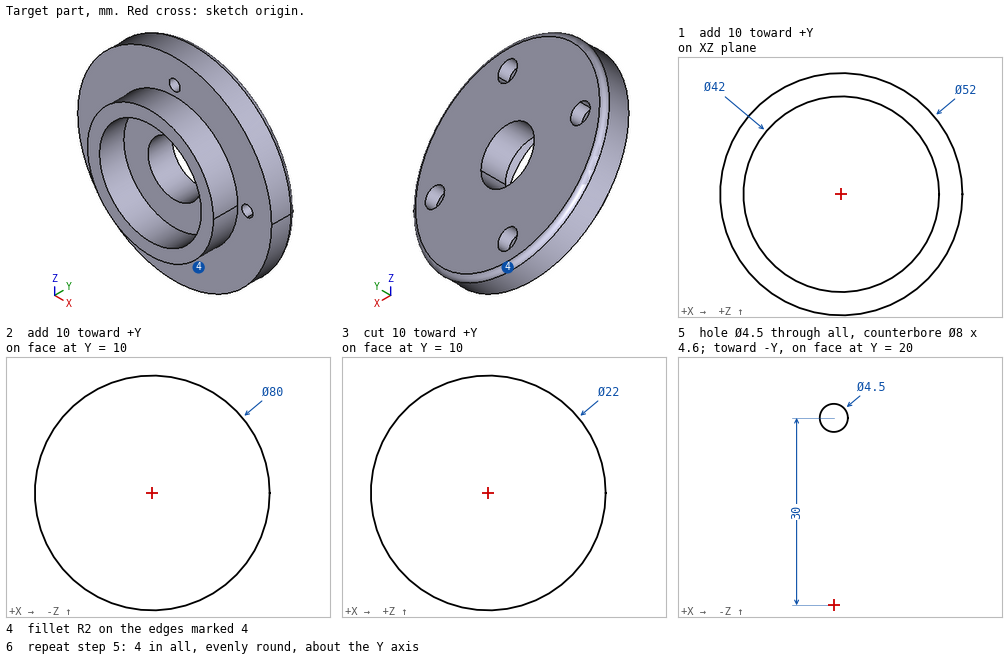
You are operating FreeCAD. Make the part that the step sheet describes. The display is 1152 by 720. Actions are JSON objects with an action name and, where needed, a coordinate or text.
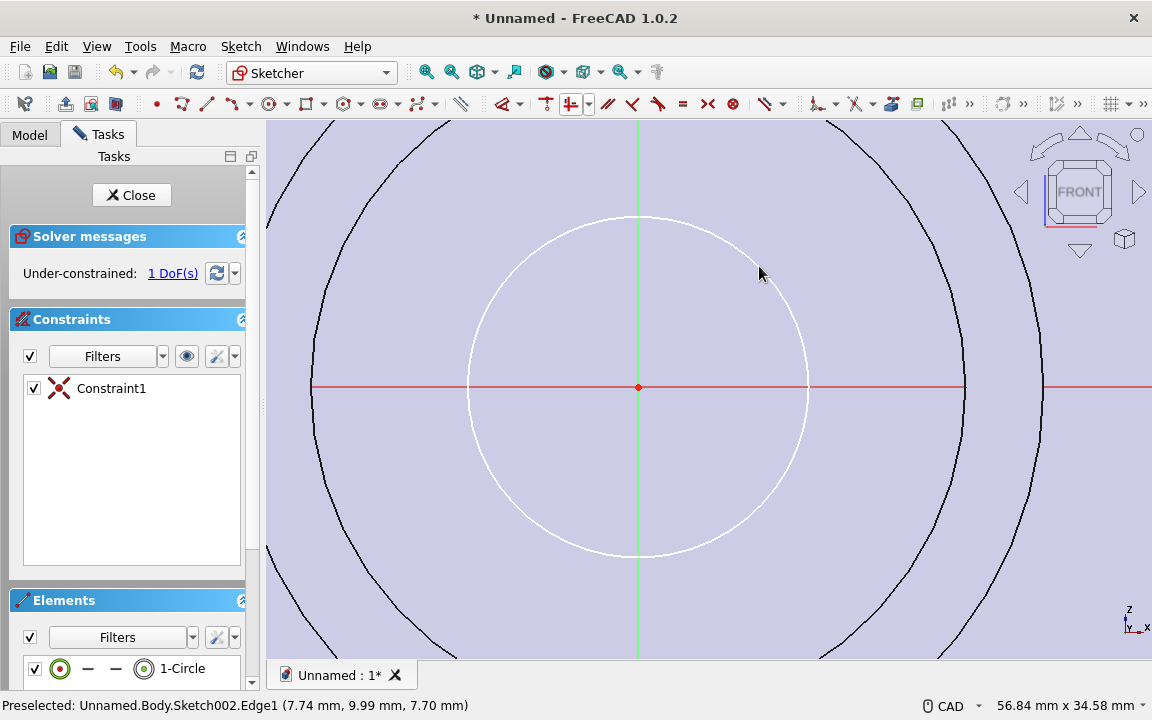
{"action": "key", "text": "d"}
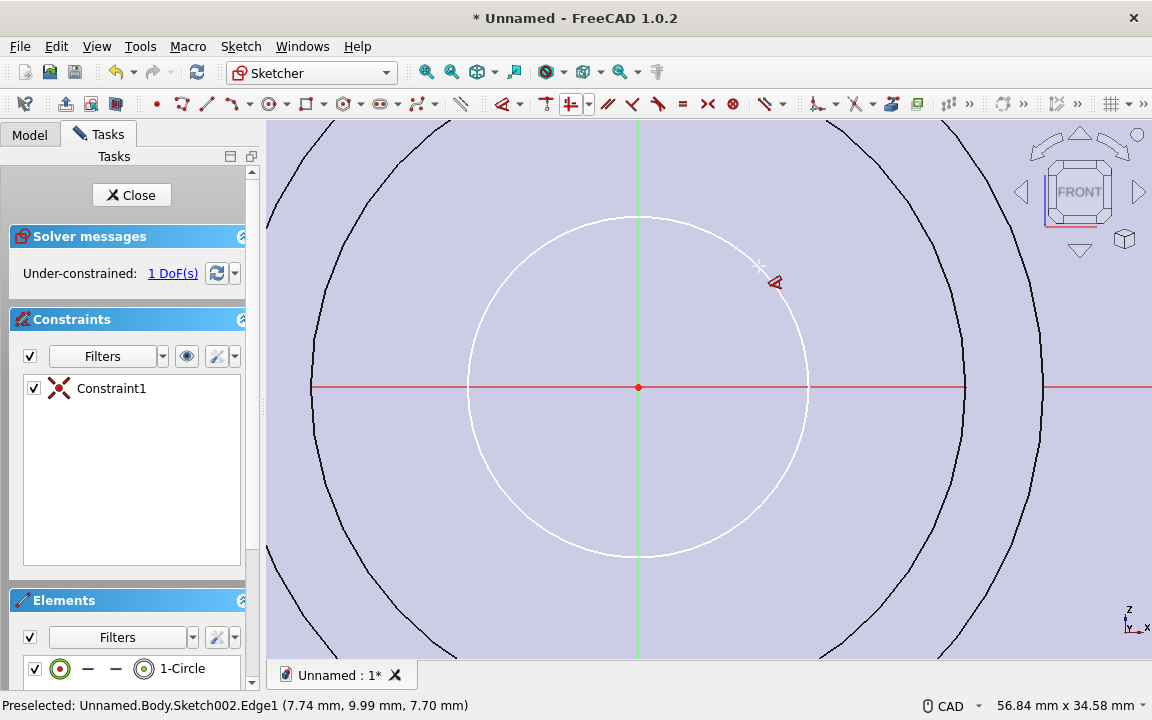
{"action": "left_click", "coordinate": [758, 266]}
{"action": "left_click", "coordinate": [781, 243]}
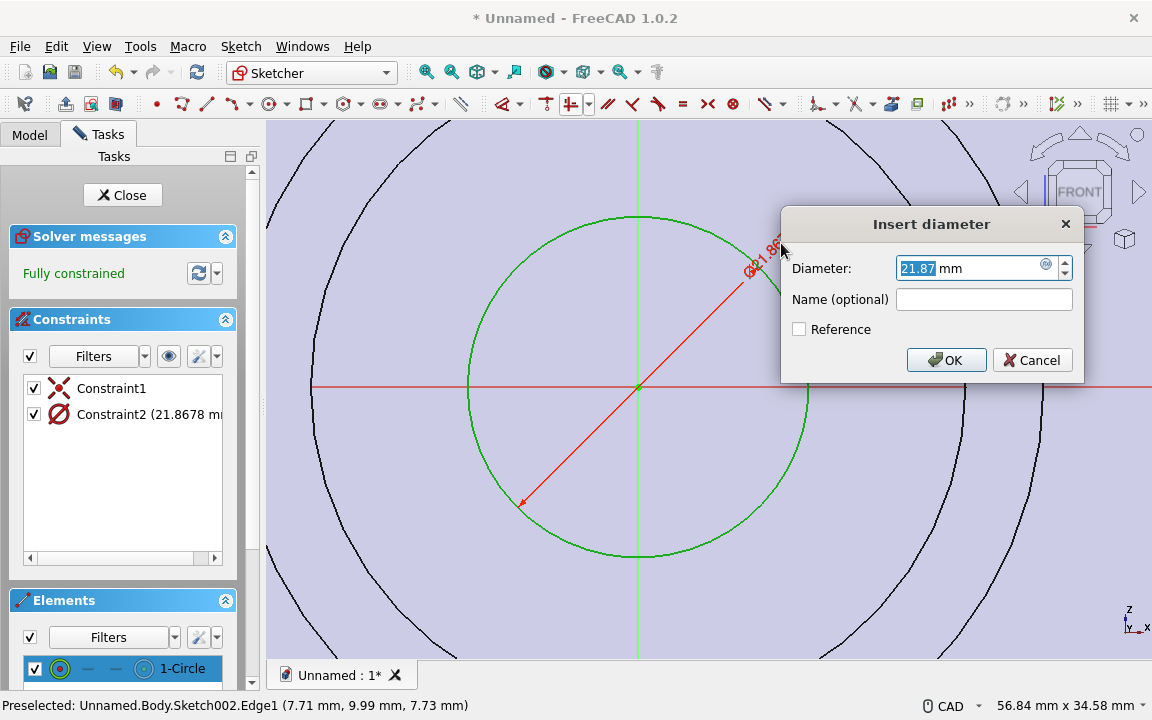
{"action": "type", "text": "22"}
{"action": "key", "text": "Return"}
{"action": "key", "text": "Escape"}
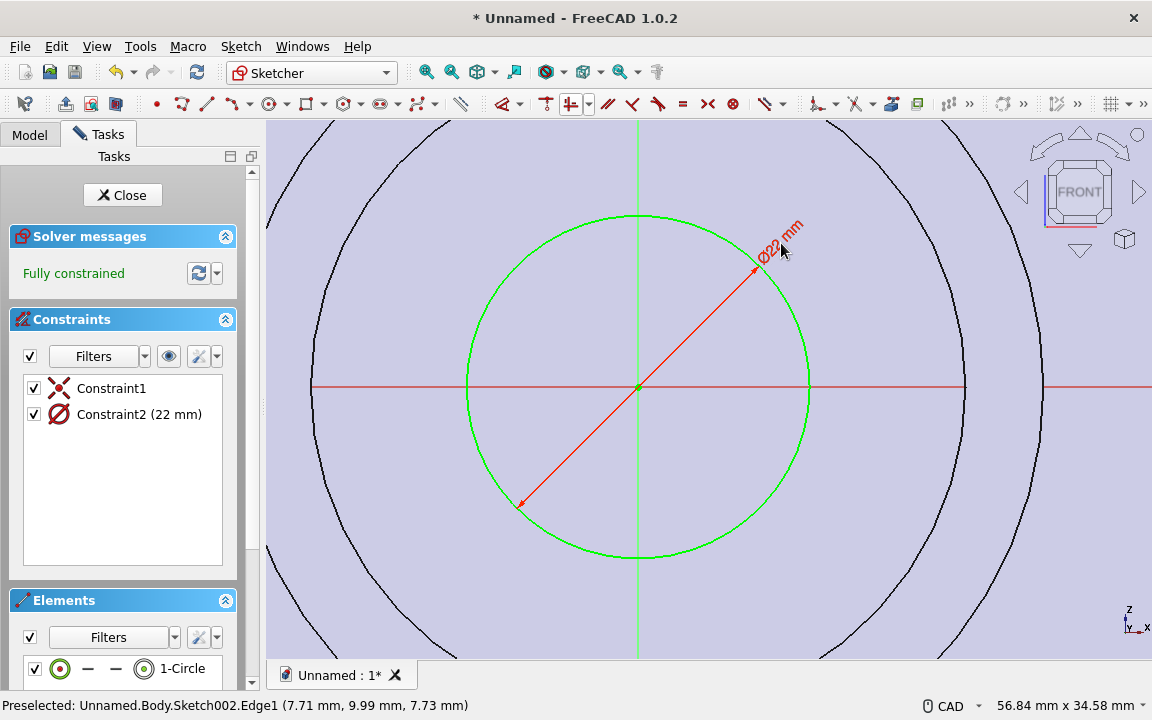
{"action": "left_click", "coordinate": [123, 195]}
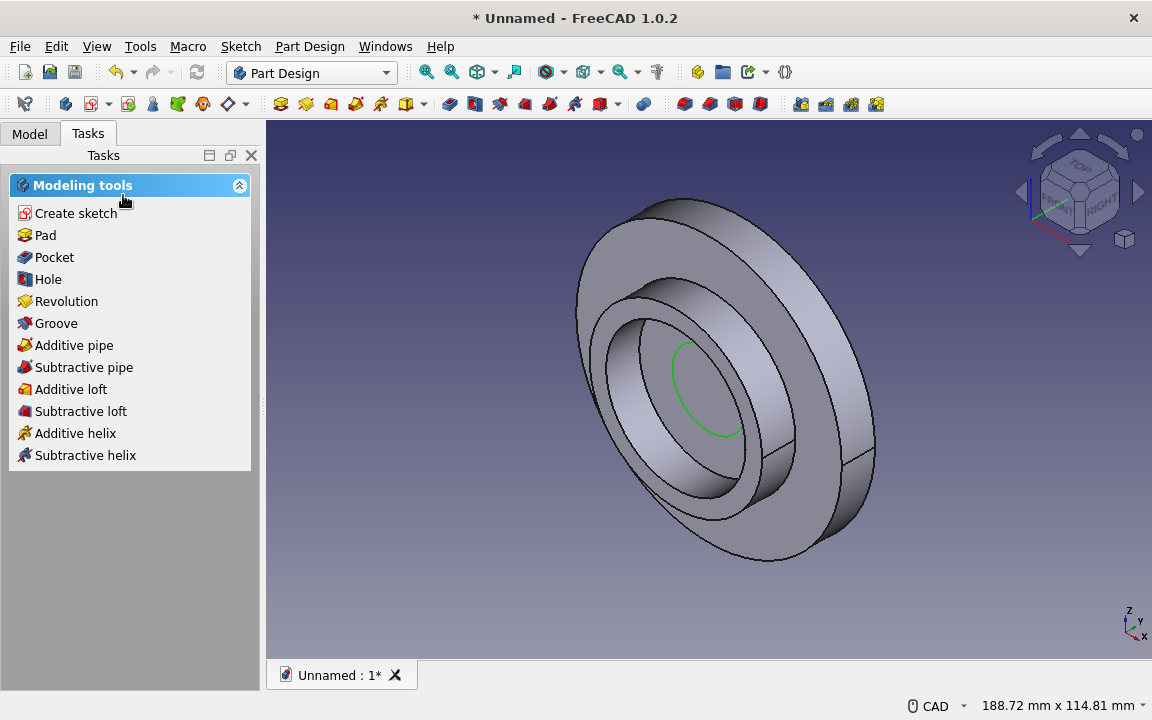
{"action": "left_click", "coordinate": [450, 104]}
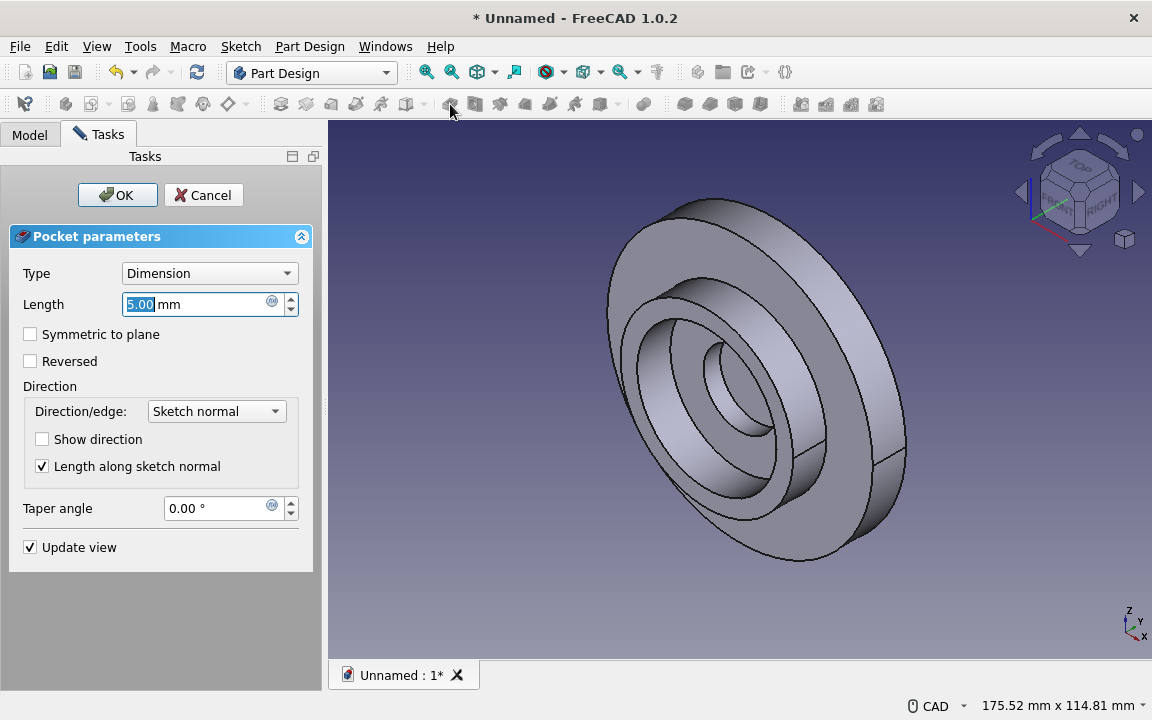
{"action": "type", "text": "10"}
{"action": "key", "text": "Tab"}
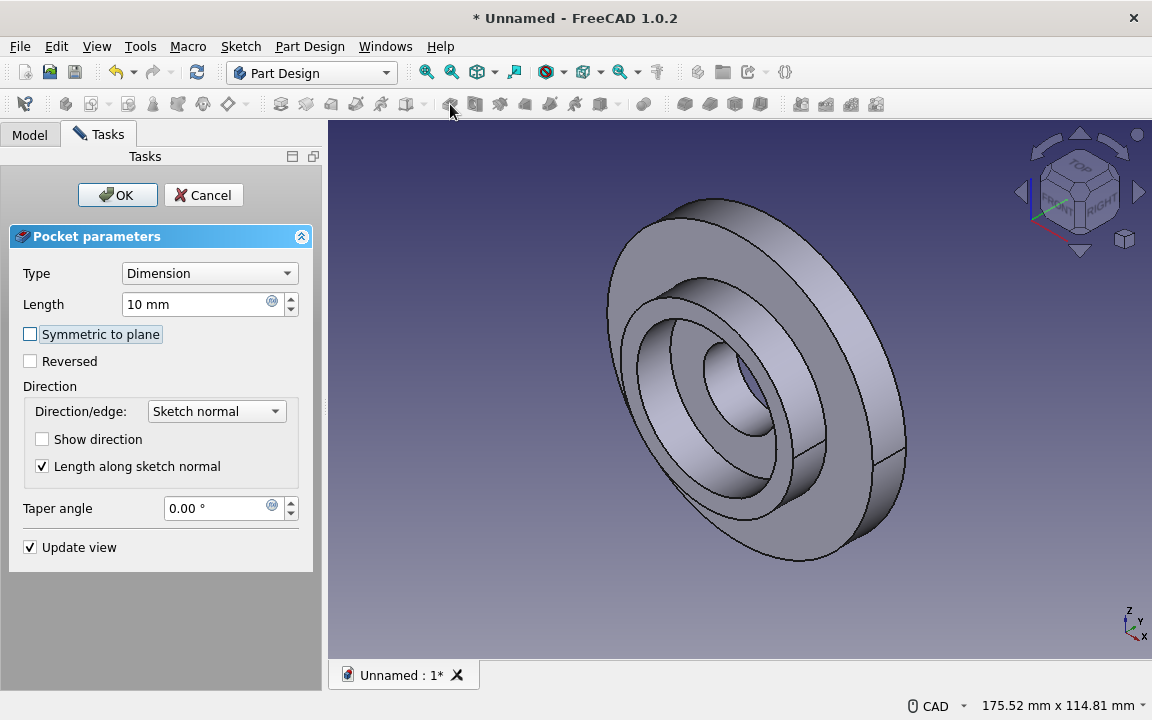
{"action": "left_click", "coordinate": [118, 195]}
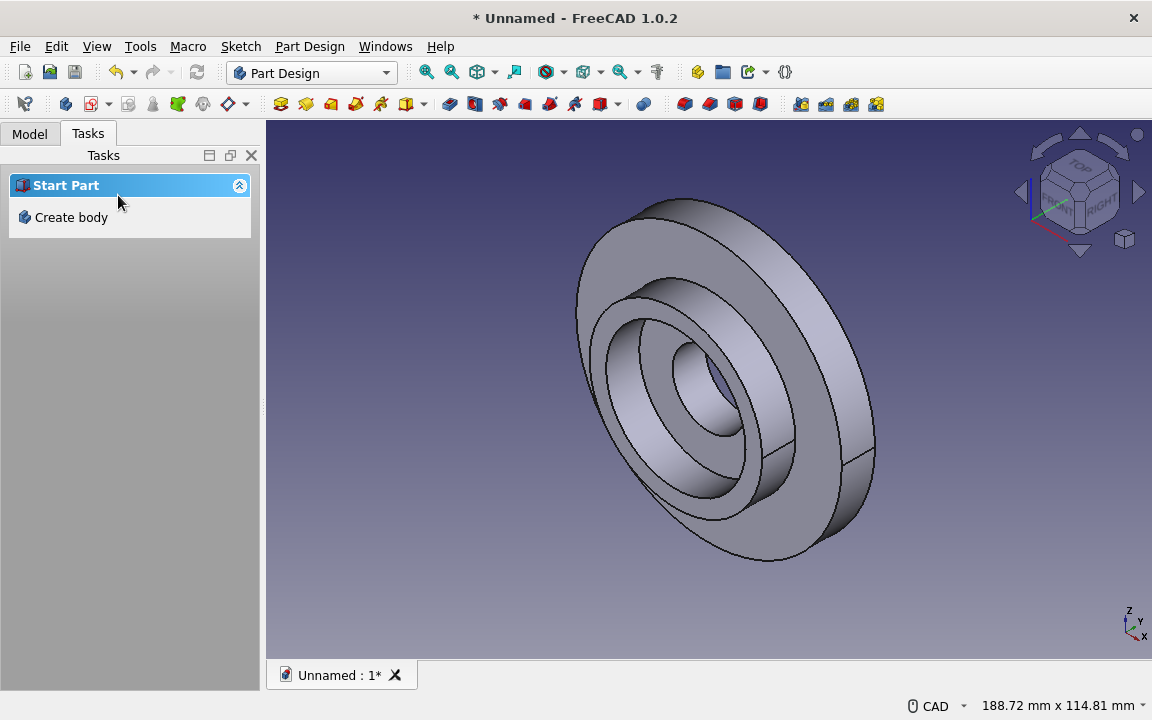
{"action": "key", "text": "2"}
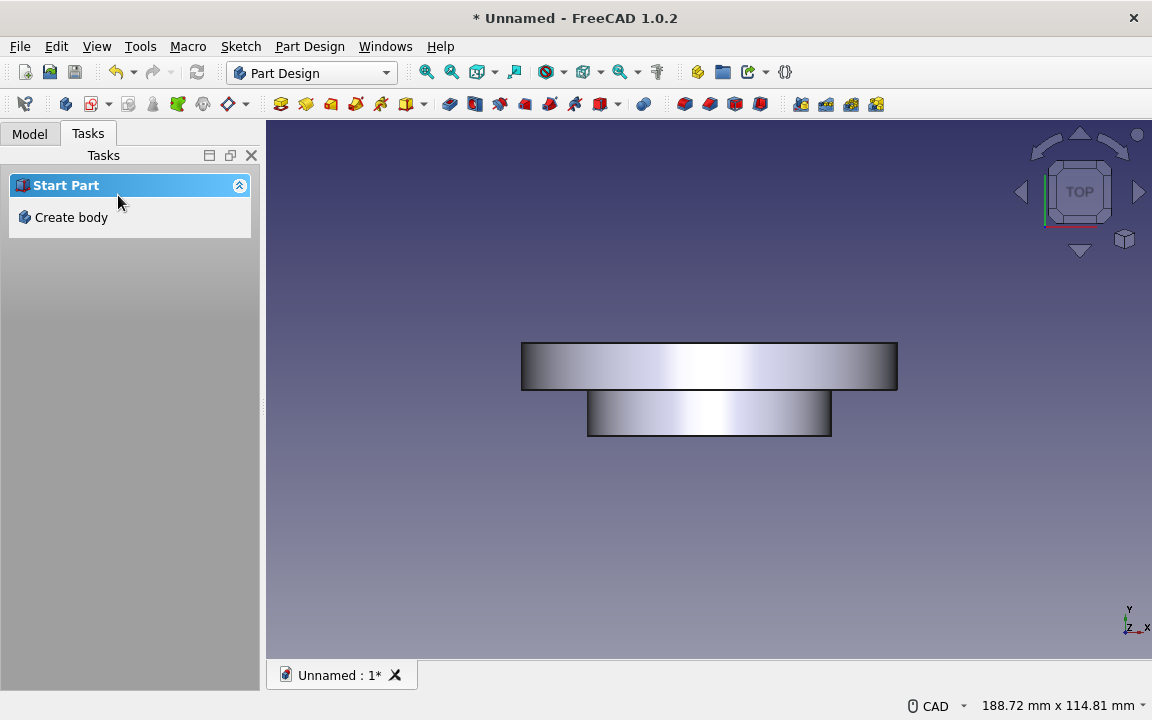
{"action": "left_click", "coordinate": [427, 72]}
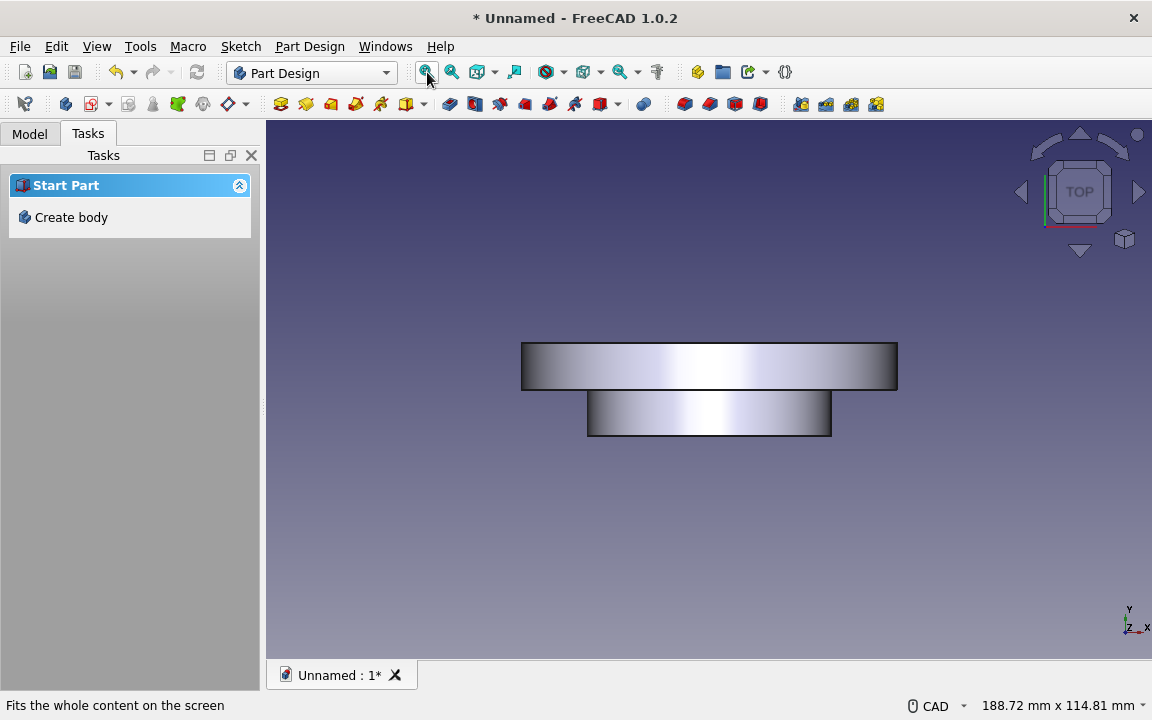
{"action": "left_click", "coordinate": [557, 342]}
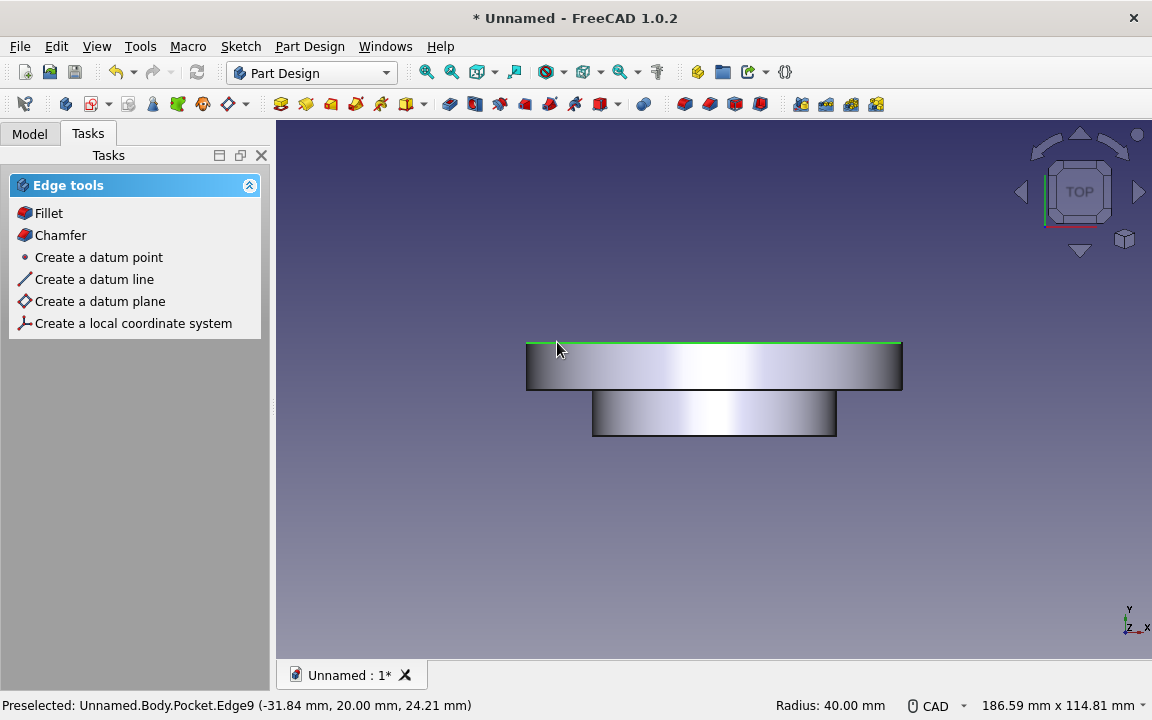
{"action": "left_click", "coordinate": [685, 104]}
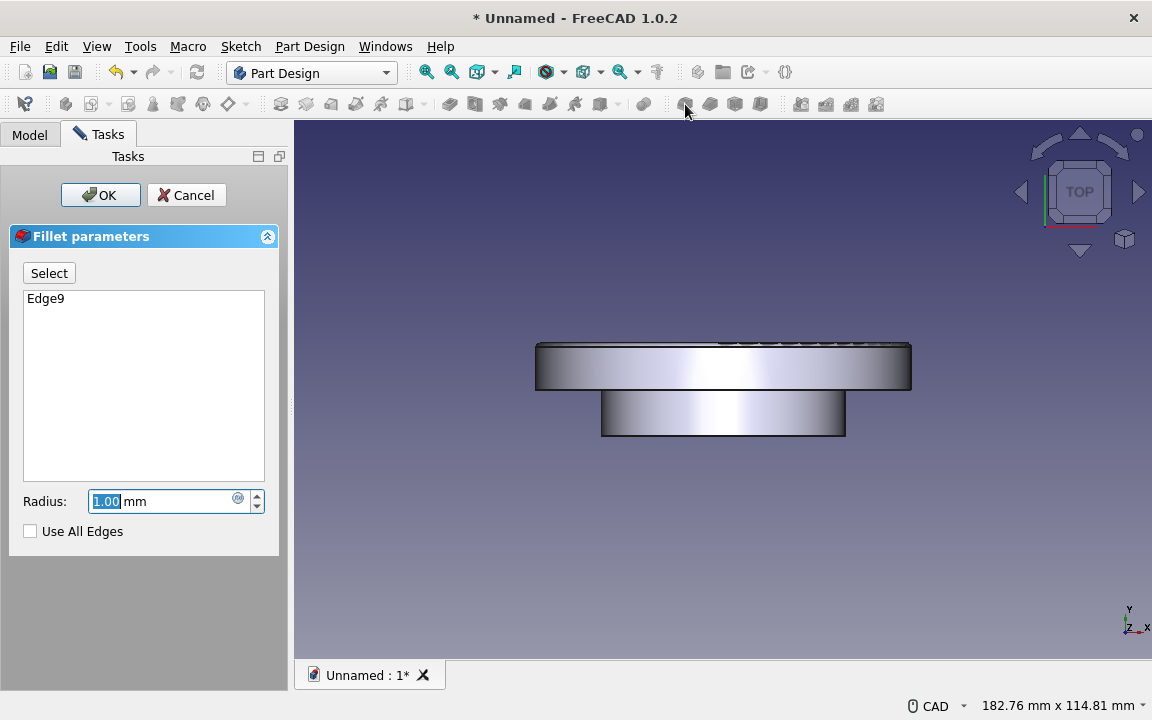
{"action": "type", "text": "2"}
{"action": "key", "text": "Tab"}